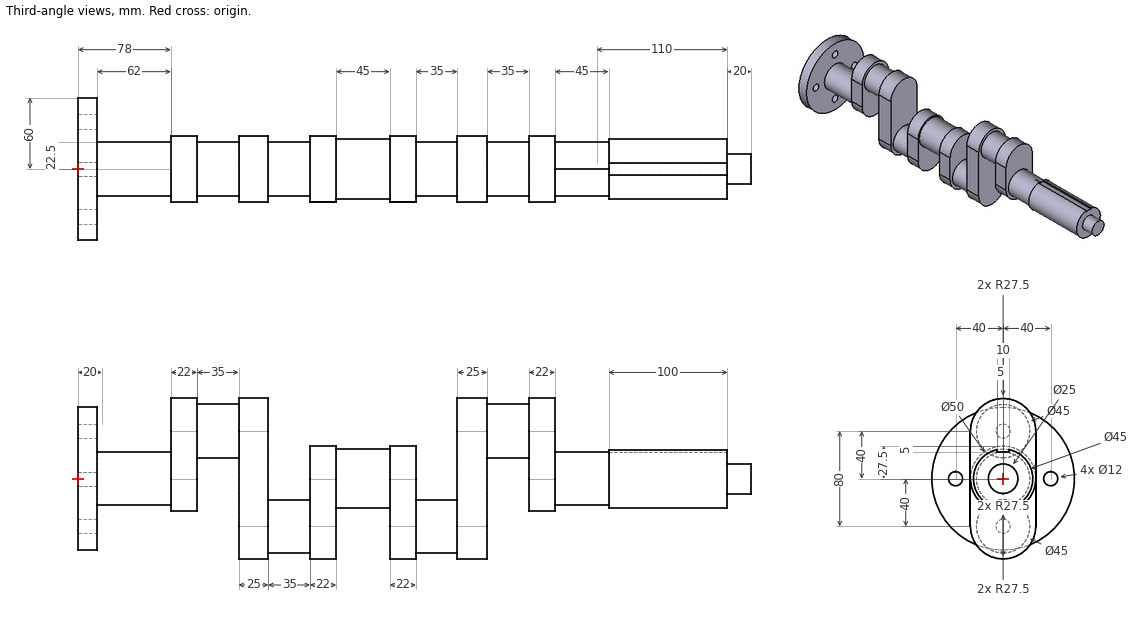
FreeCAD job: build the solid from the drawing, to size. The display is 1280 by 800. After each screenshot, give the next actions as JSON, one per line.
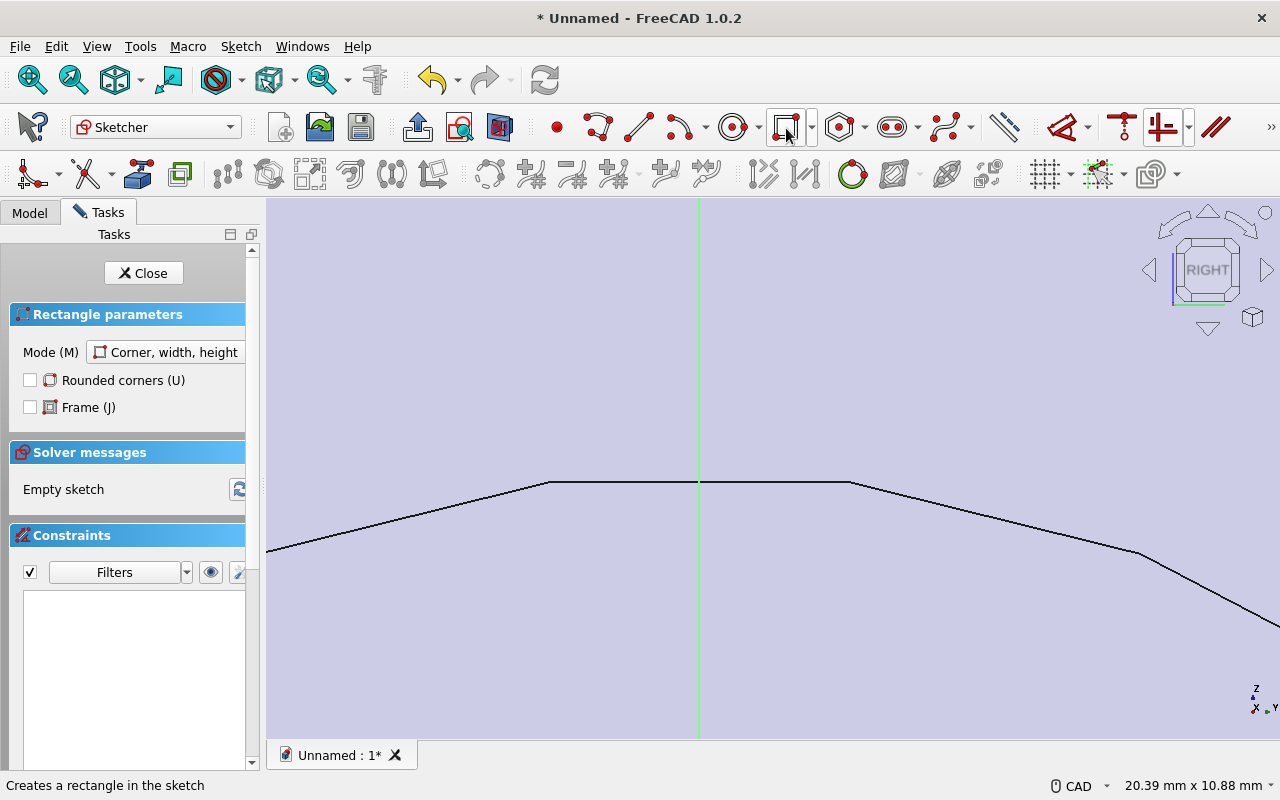
{"action": "left_click", "coordinate": [451, 349]}
{"action": "left_click", "coordinate": [948, 597]}
{"action": "key", "text": "Escape"}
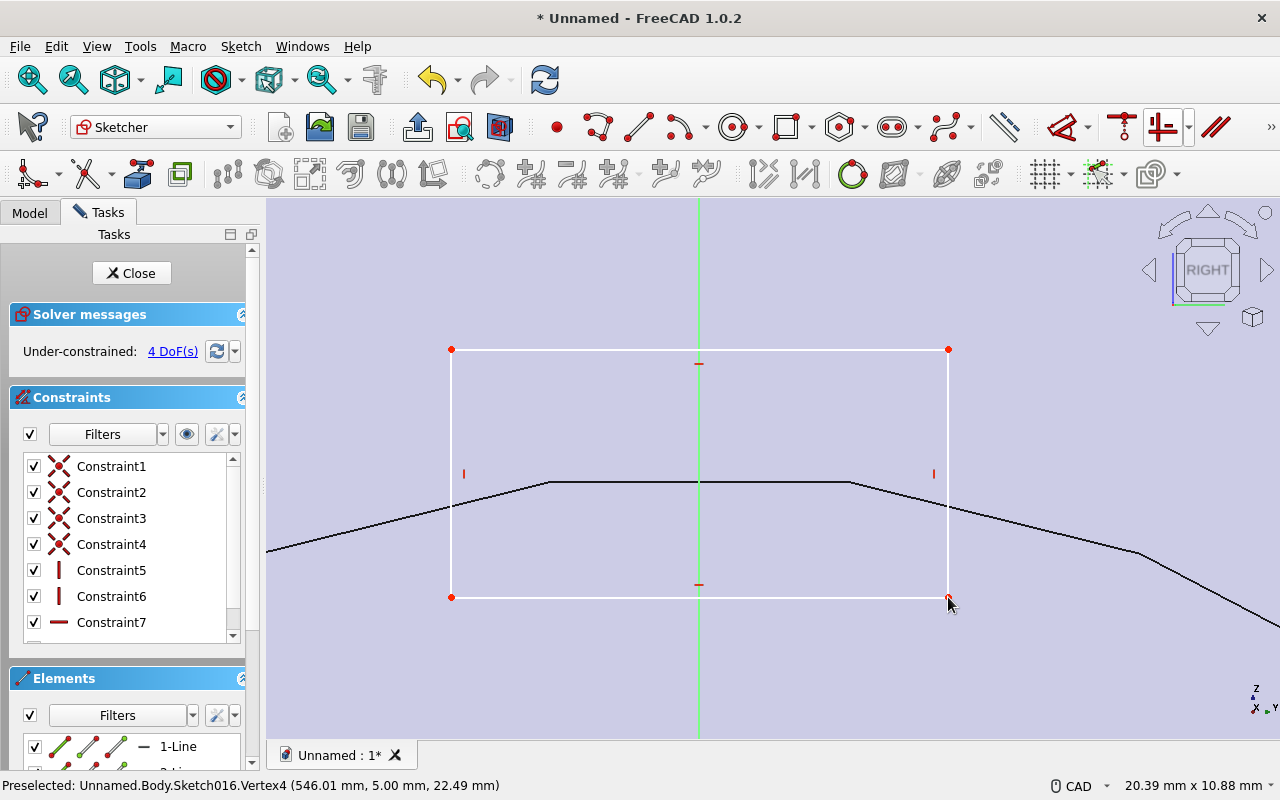
{"action": "left_click", "coordinate": [1062, 128]}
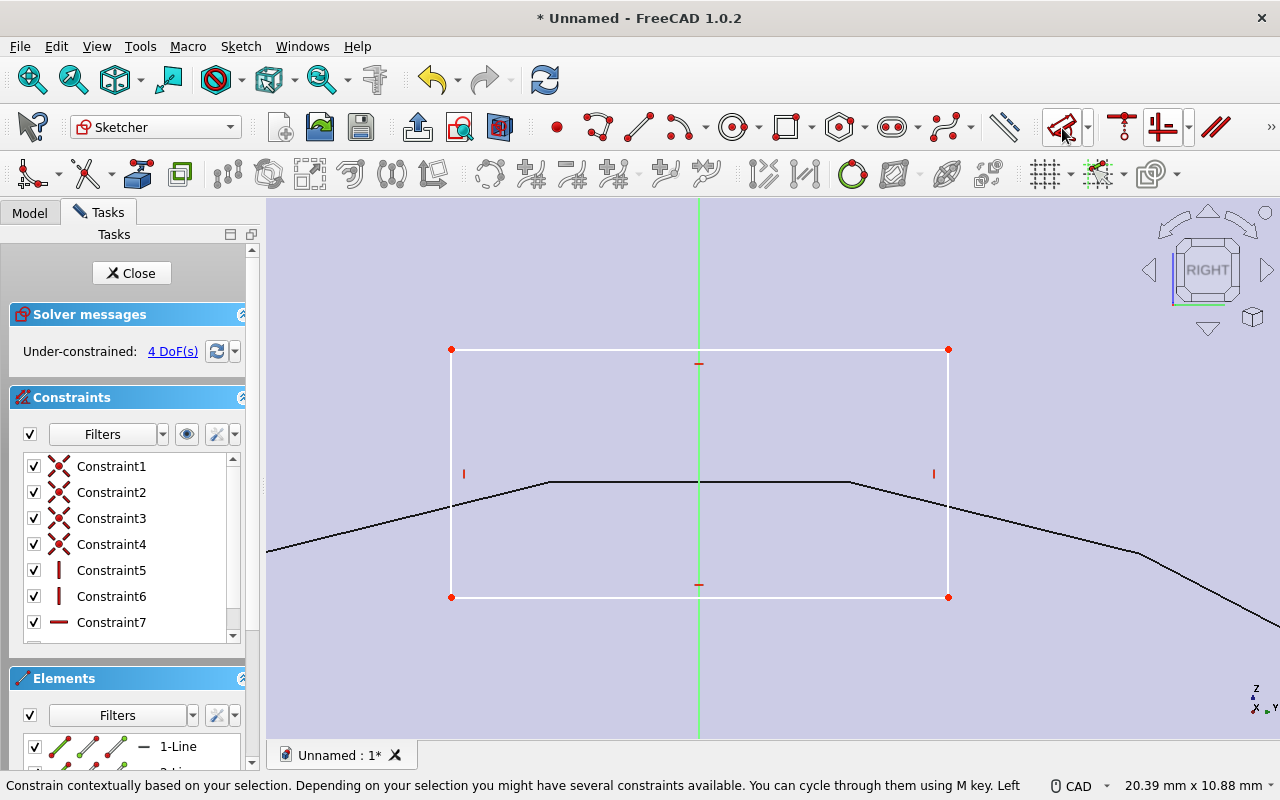
{"action": "left_click", "coordinate": [451, 424]}
{"action": "left_click", "coordinate": [417, 474]}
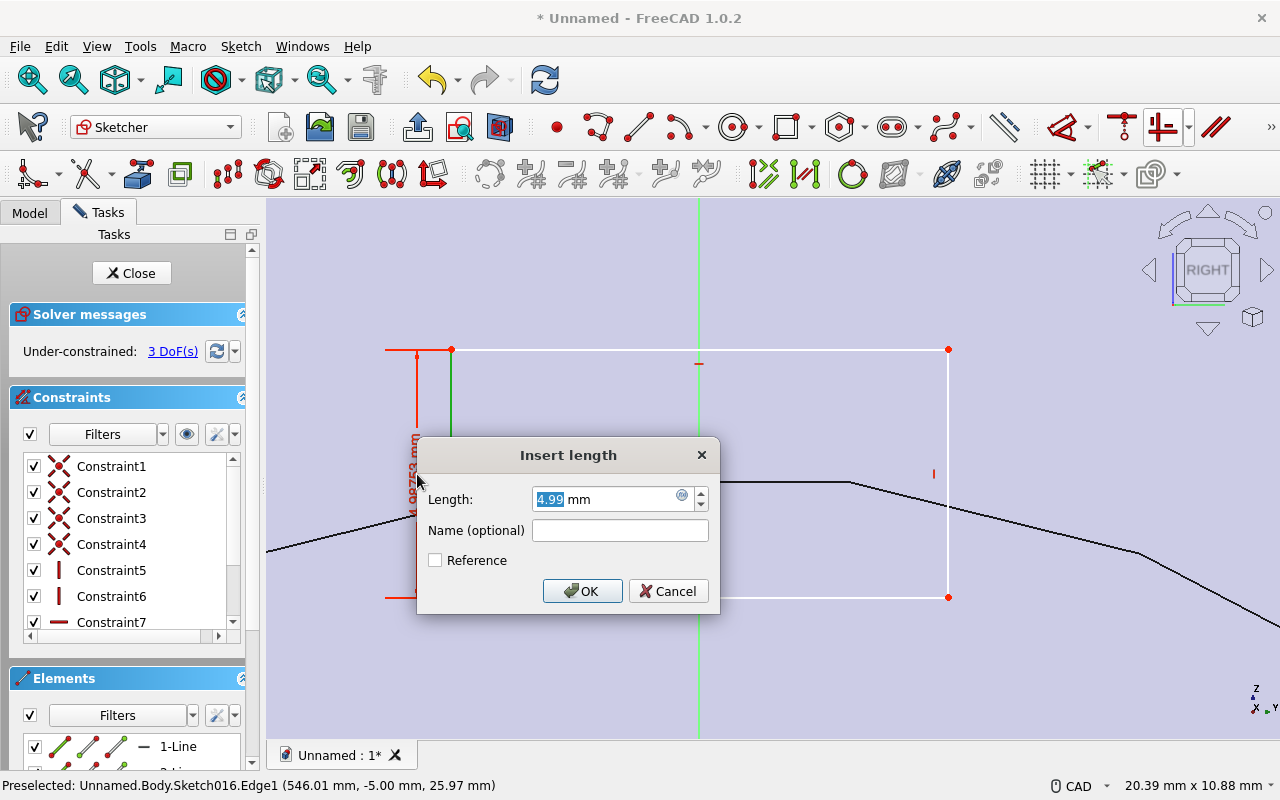
{"action": "type", "text": "5"}
{"action": "key", "text": "Return"}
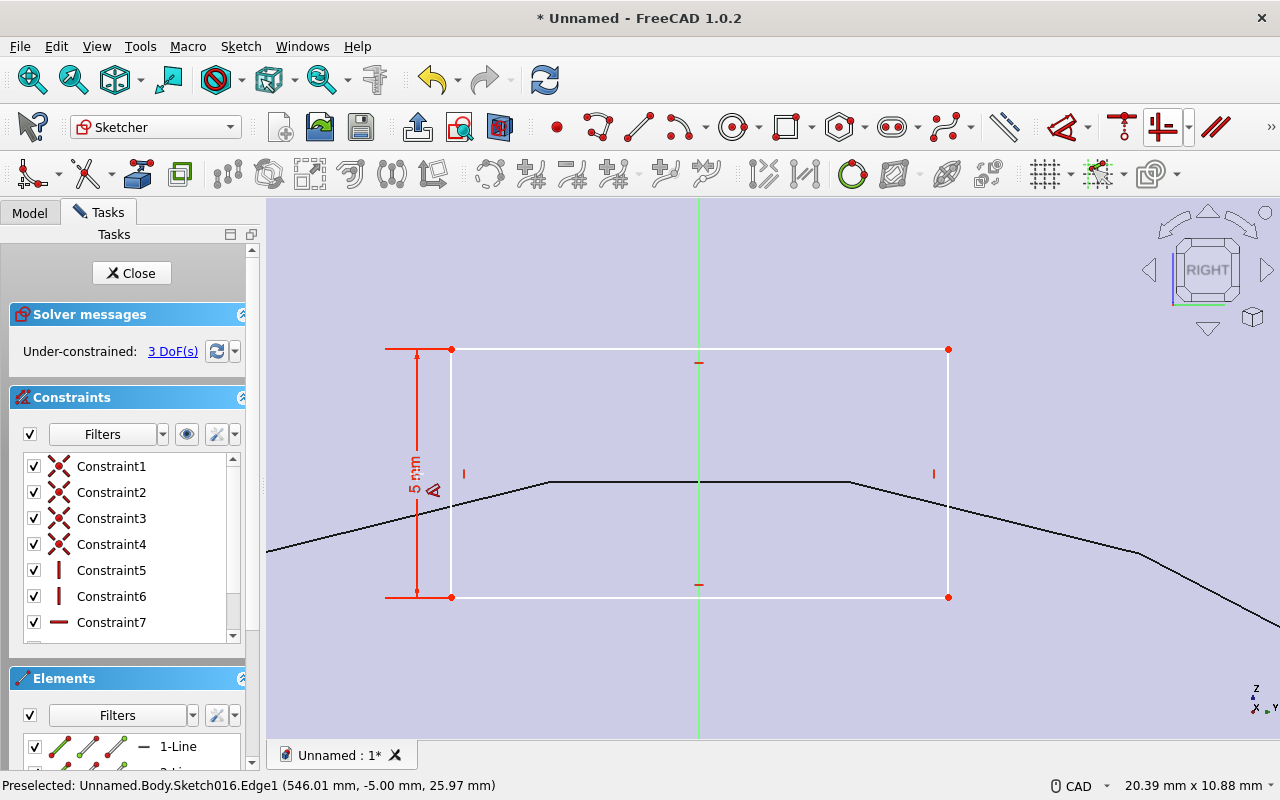
{"action": "left_click", "coordinate": [600, 598]}
{"action": "left_click", "coordinate": [585, 632]}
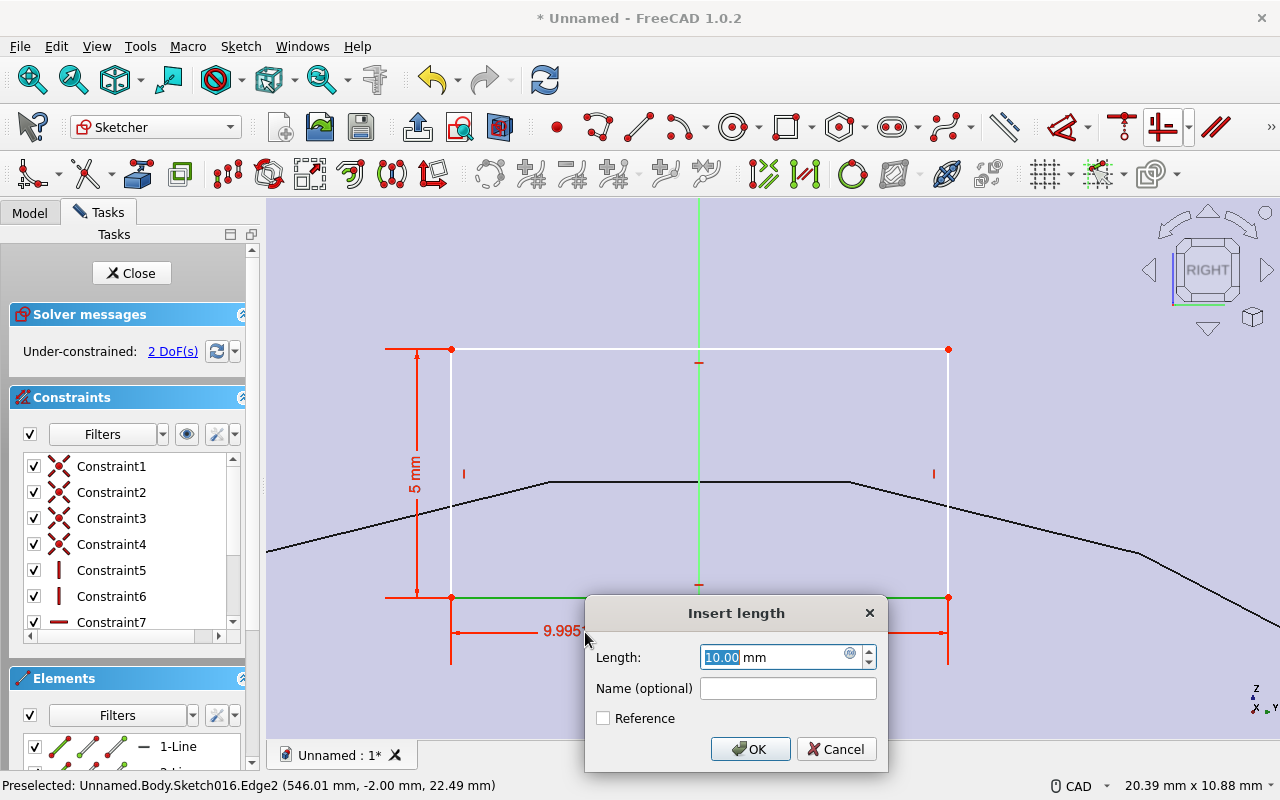
{"action": "type", "text": "10"}
{"action": "key", "text": "Return"}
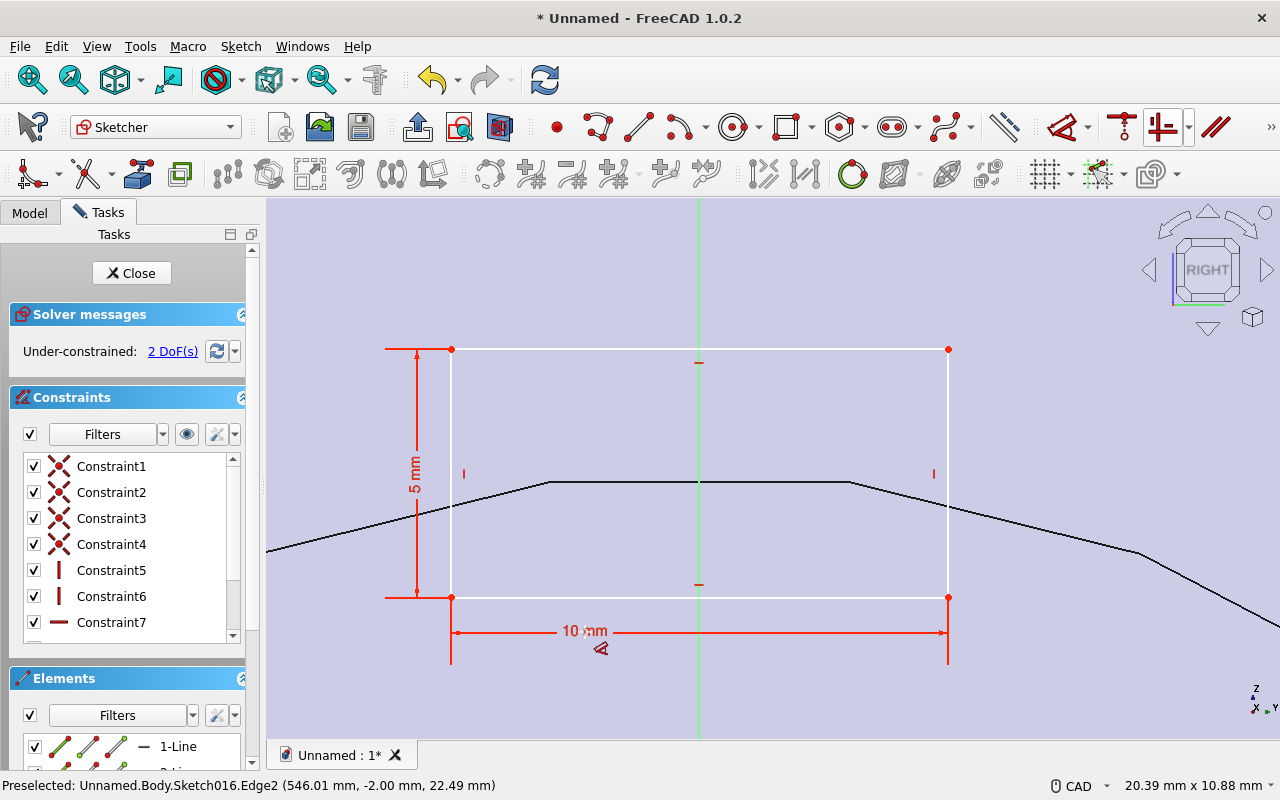
{"action": "left_click", "coordinate": [451, 349]}
{"action": "left_click", "coordinate": [575, 315]}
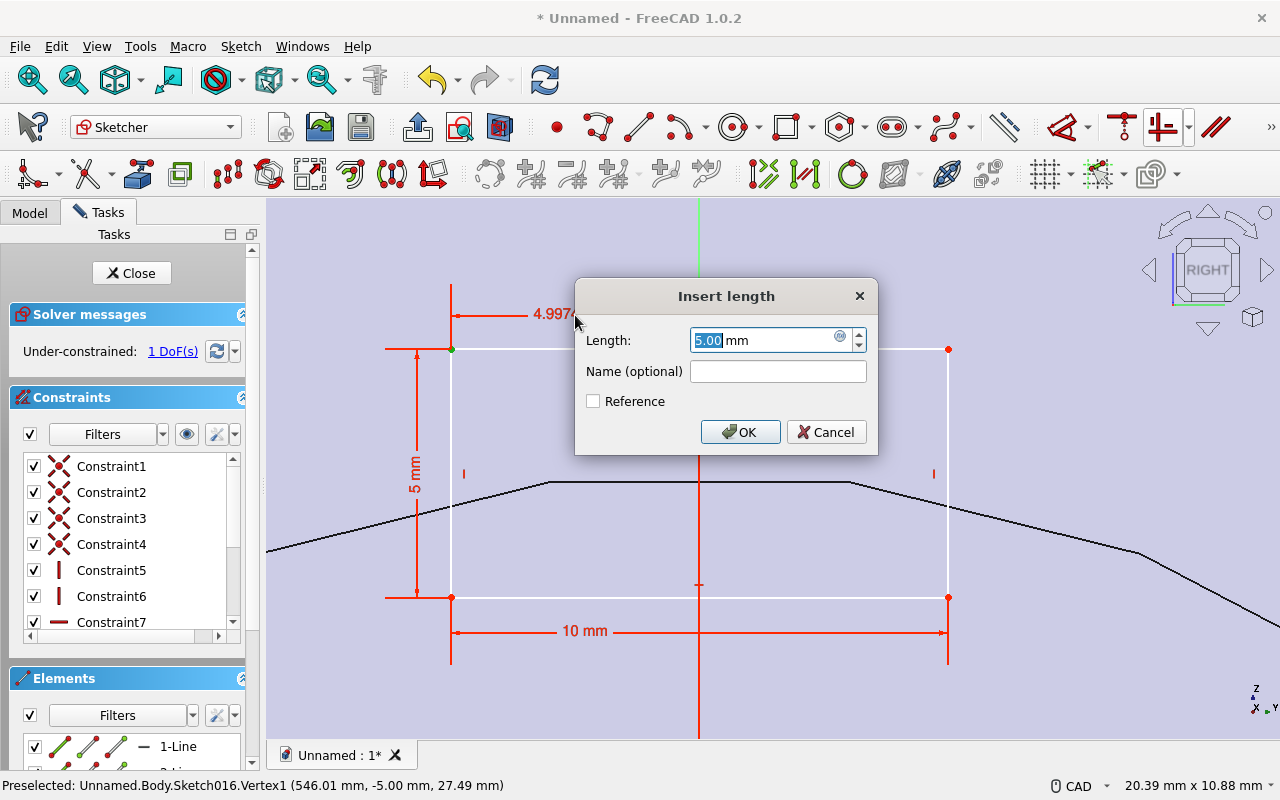
{"action": "type", "text": "5"}
{"action": "key", "text": "Return"}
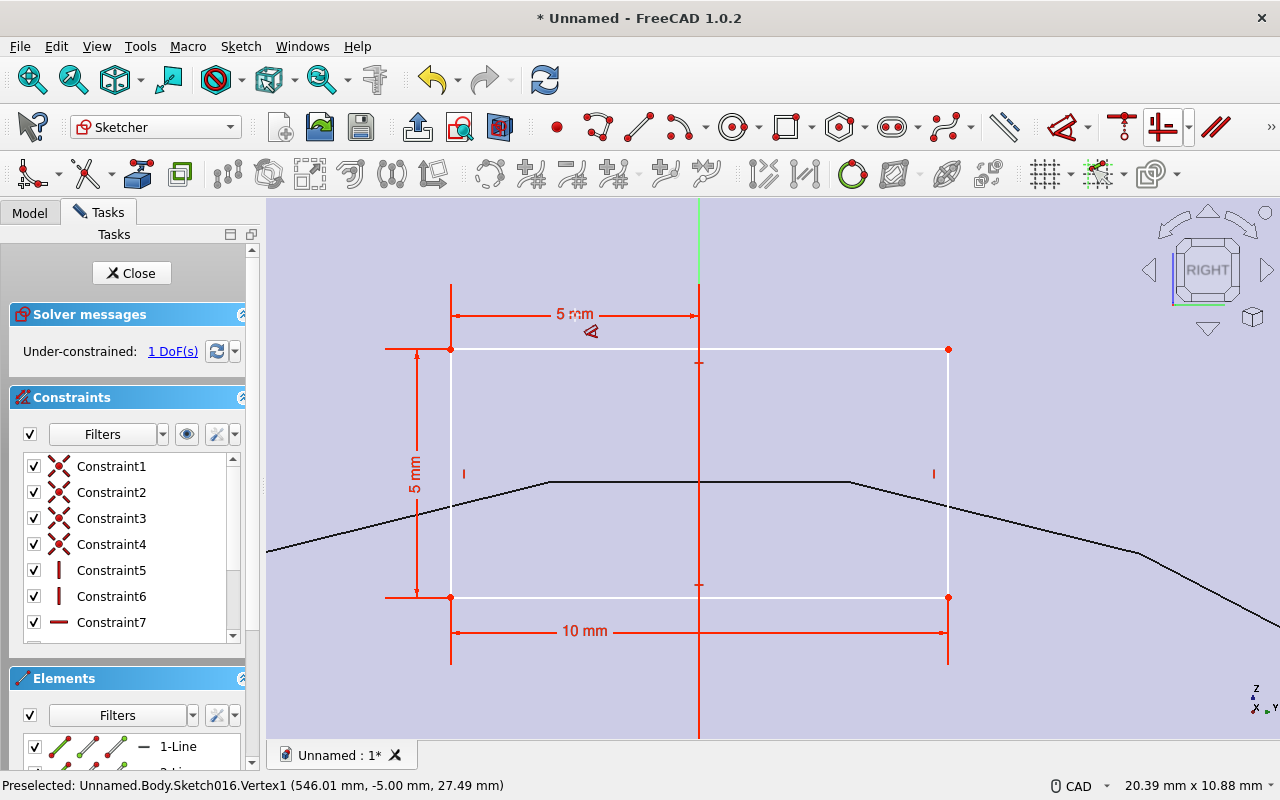
{"action": "left_click", "coordinate": [451, 349]}
{"action": "left_click", "coordinate": [417, 530]}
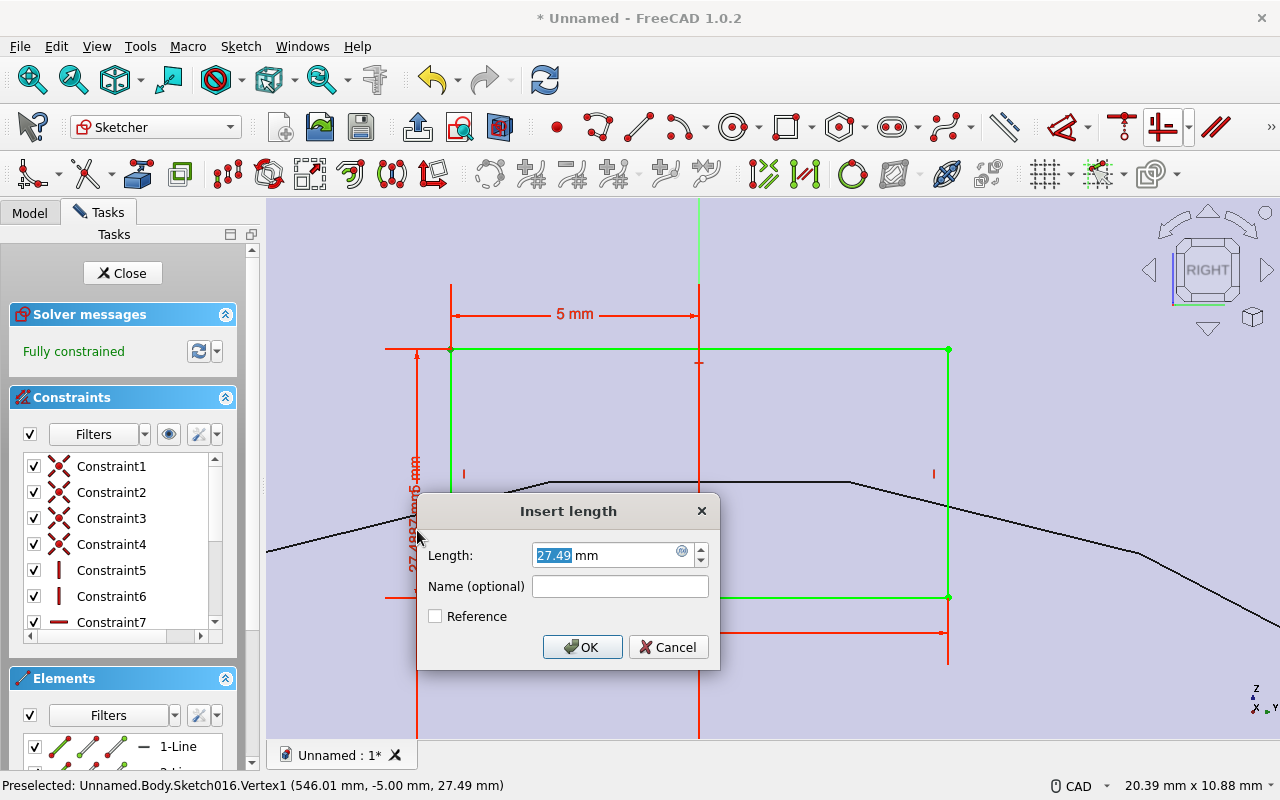
{"action": "type", "text": "27.5"}
{"action": "key", "text": "Return"}
{"action": "key", "text": "Escape"}